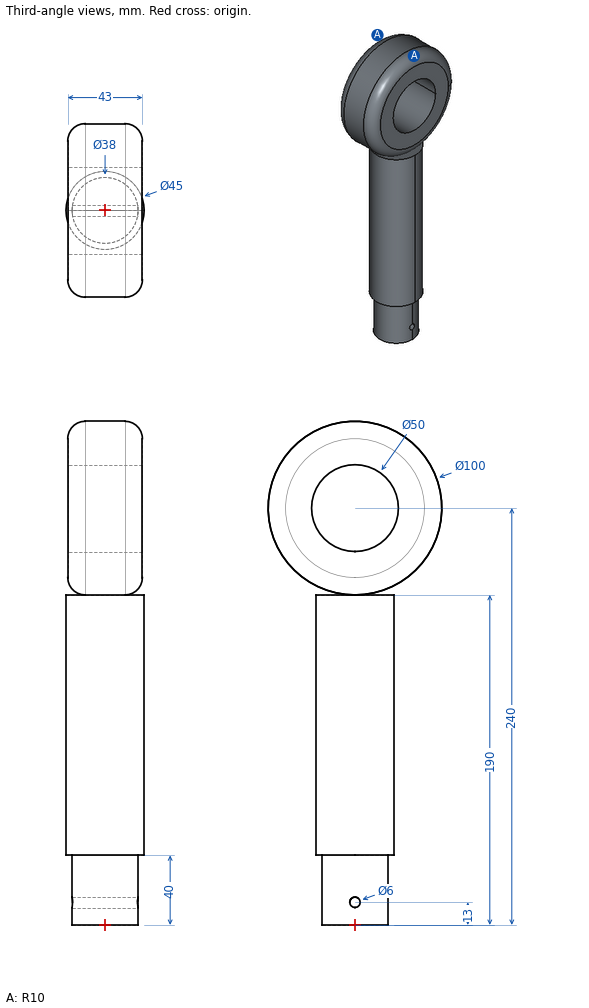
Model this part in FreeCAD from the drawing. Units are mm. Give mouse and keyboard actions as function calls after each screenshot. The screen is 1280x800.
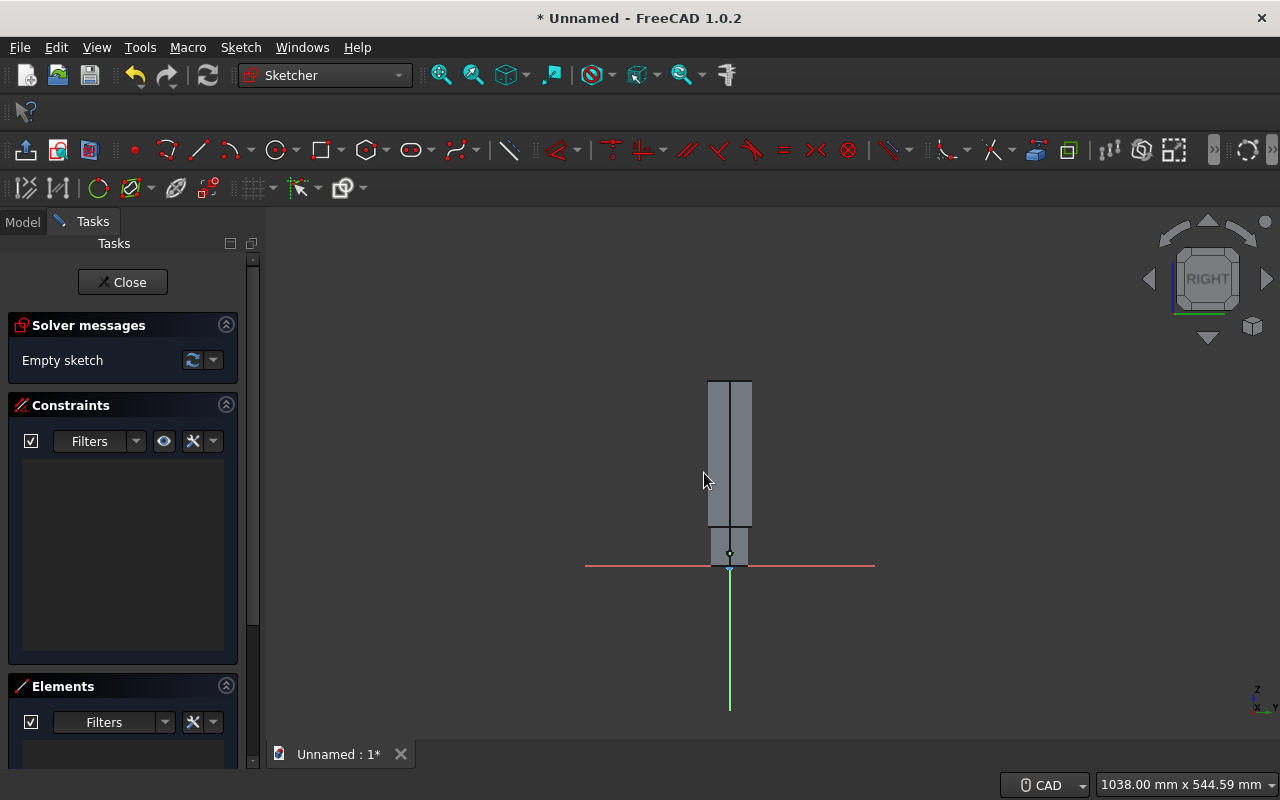
scroll(740, 271, up, 6)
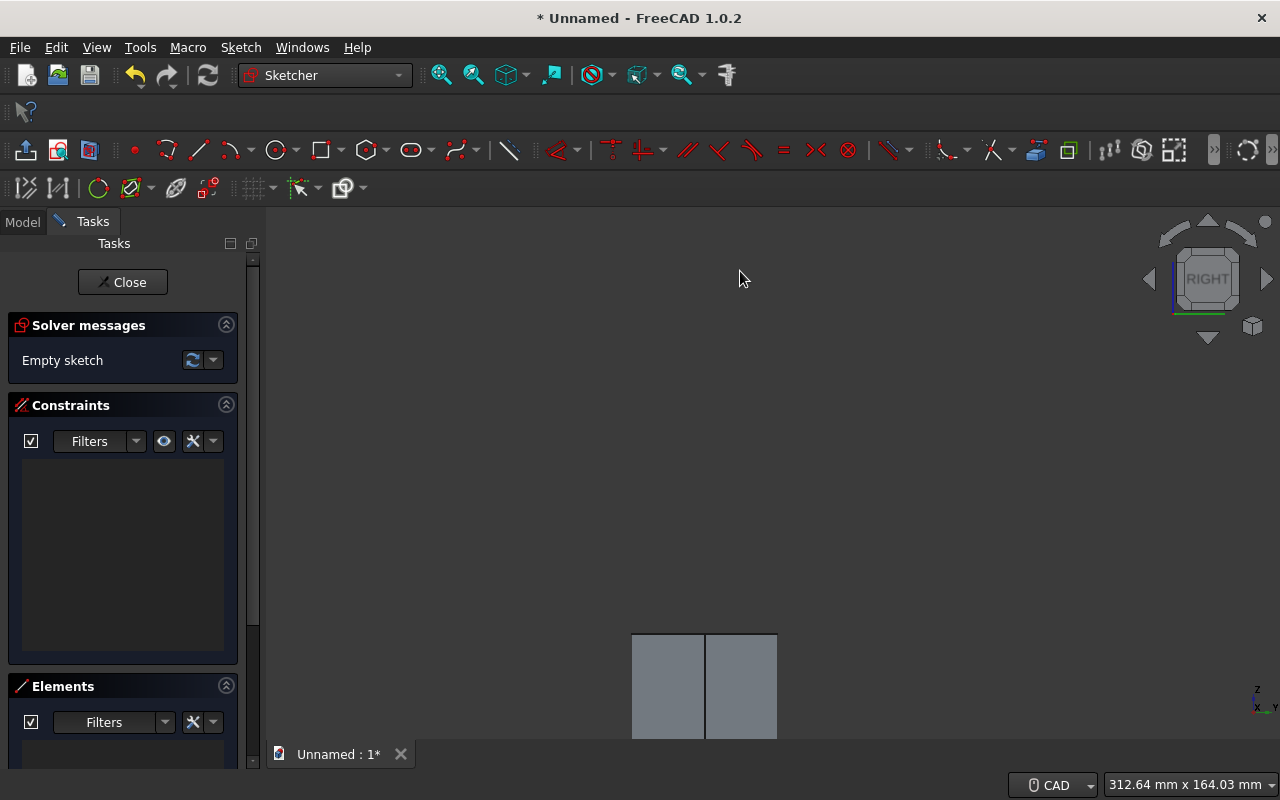
click(276, 150)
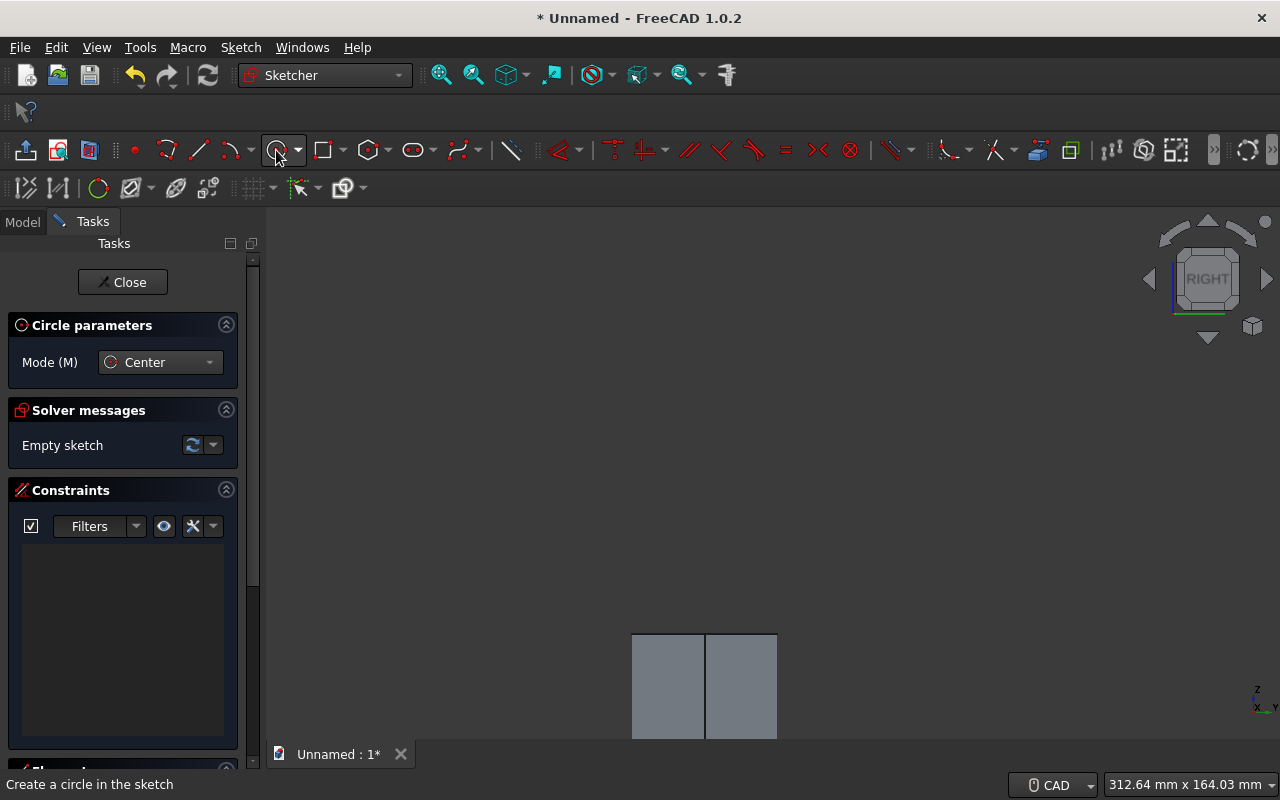
click(705, 472)
move(819, 357)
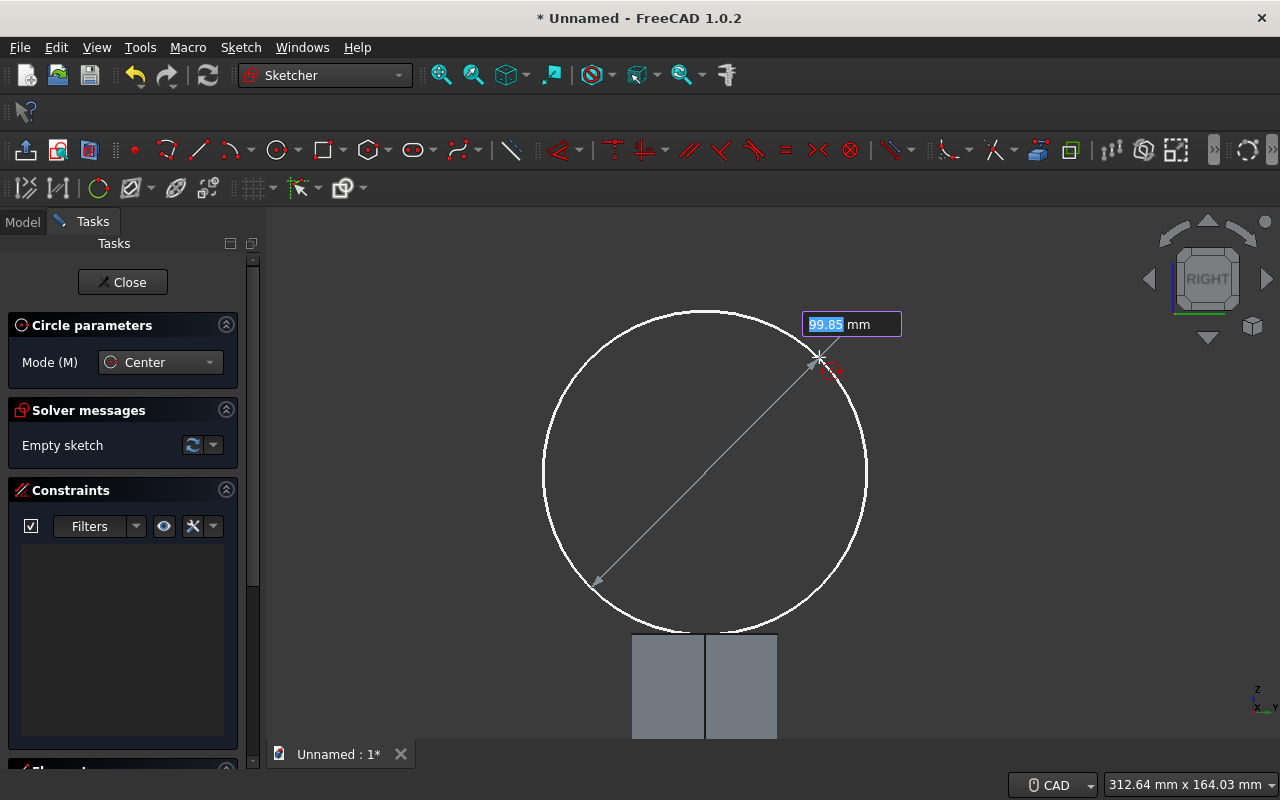
text(100)
key(Return)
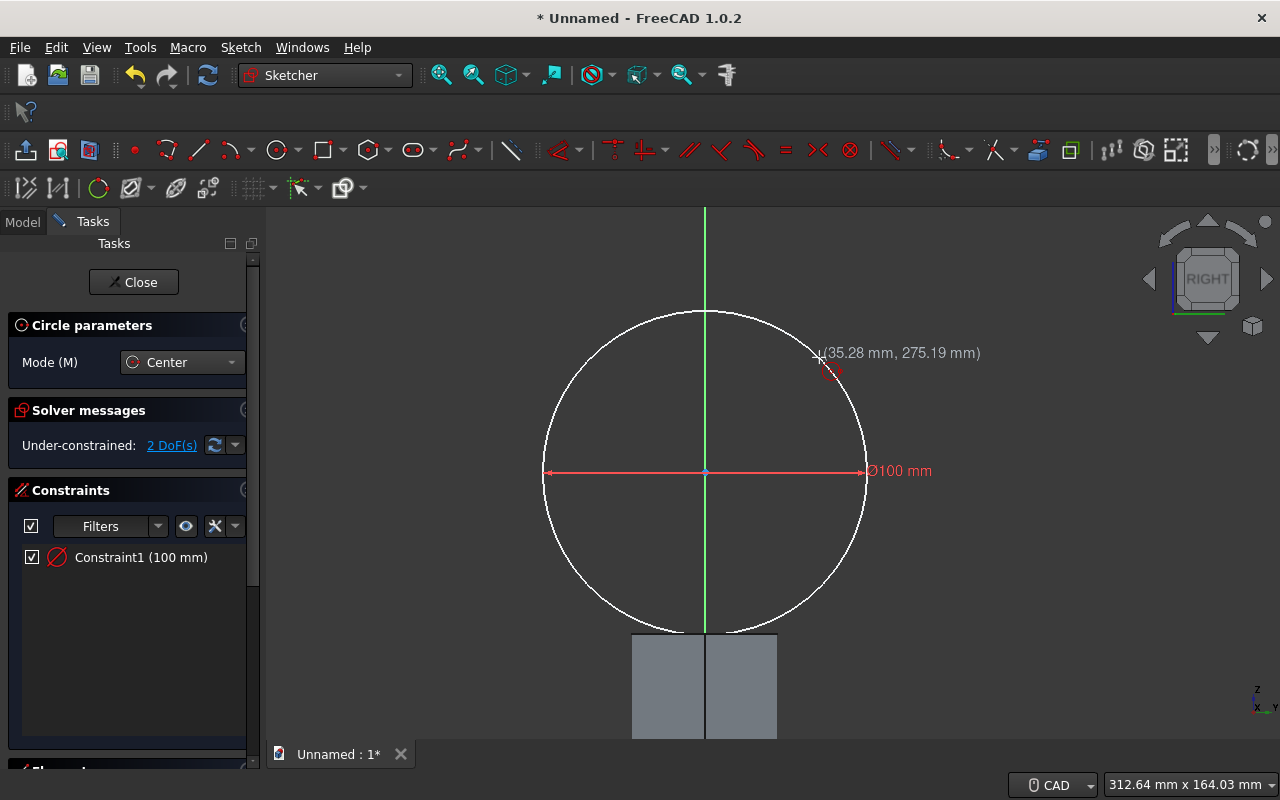
click(705, 473)
move(762, 415)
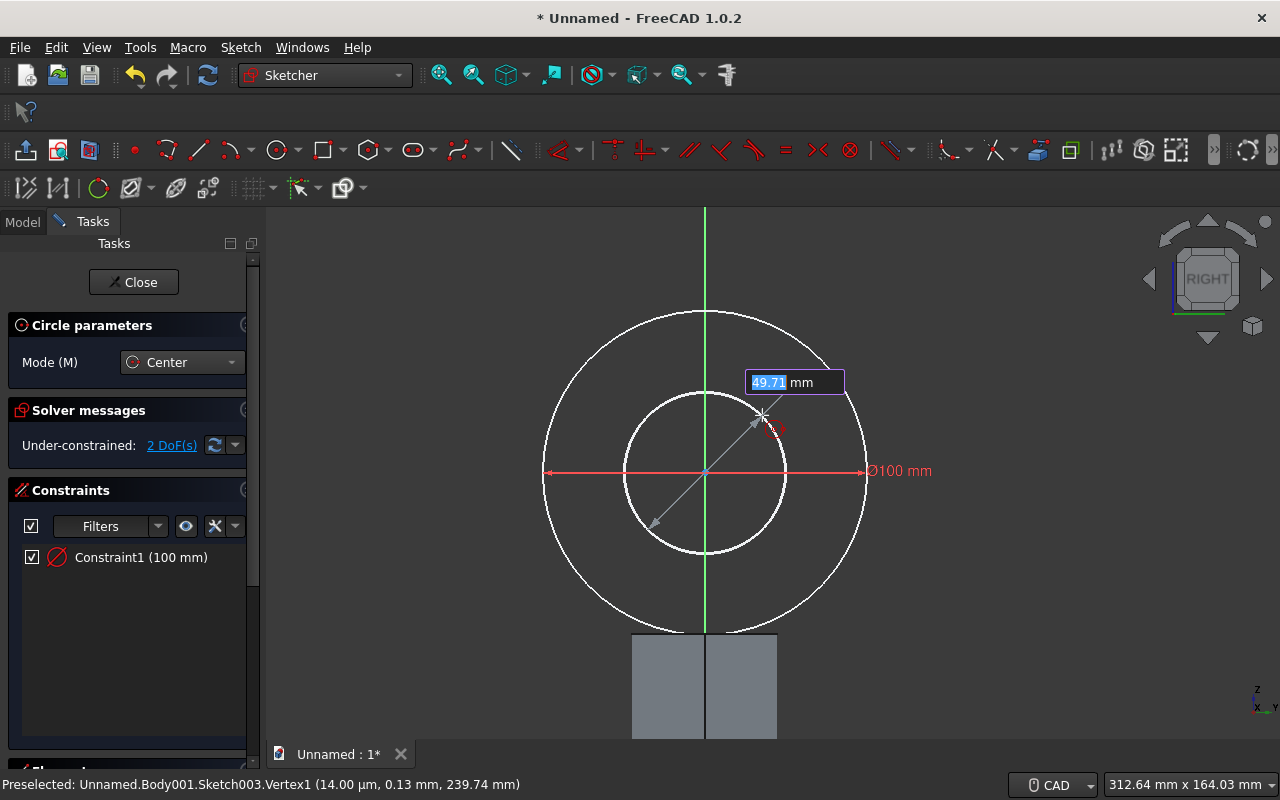
text(50)
key(Return)
key(Escape)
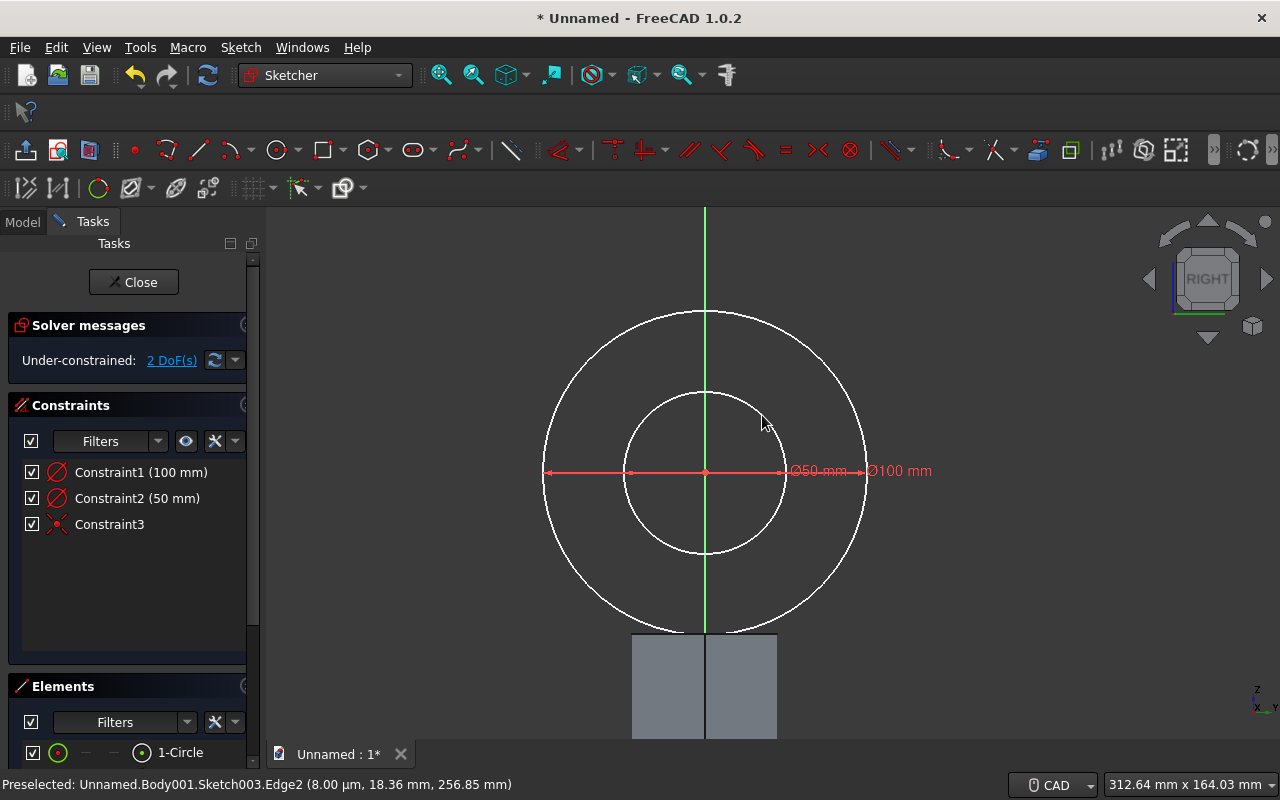
click(705, 473)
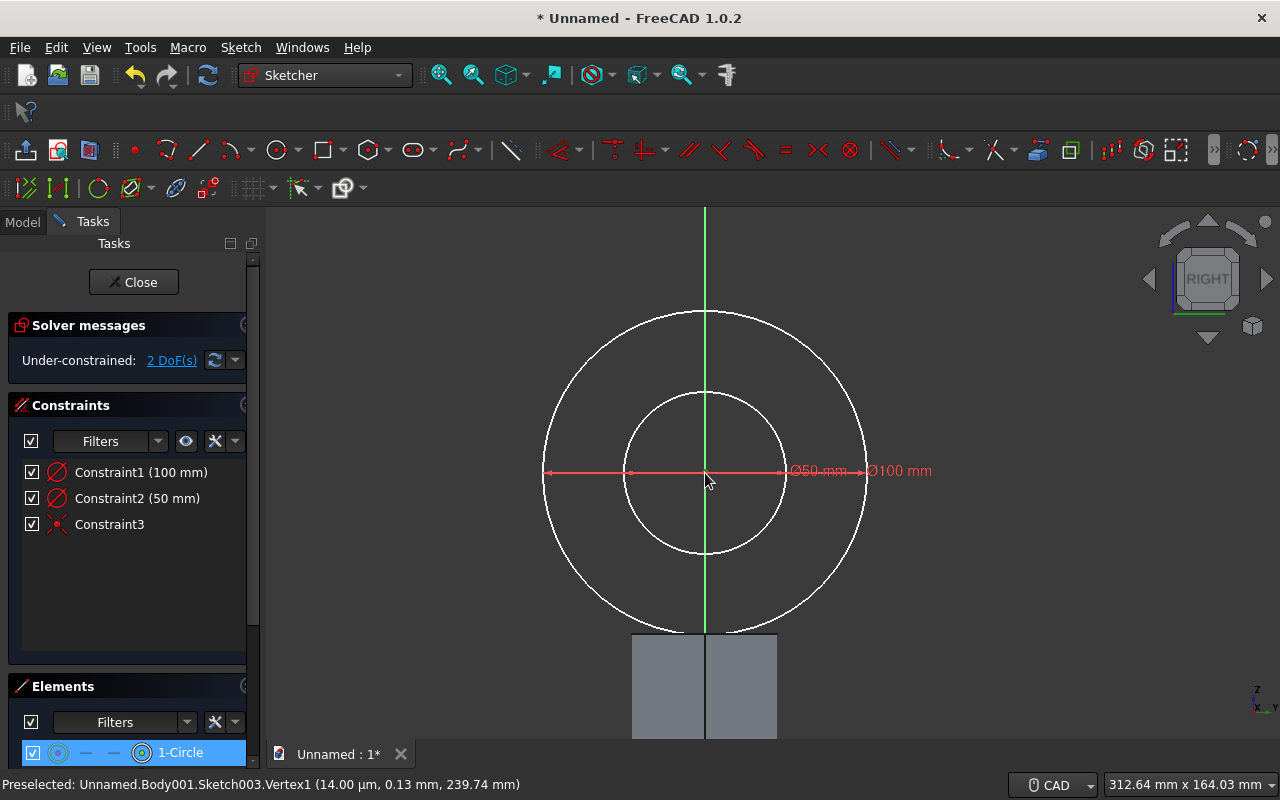
click(705, 677)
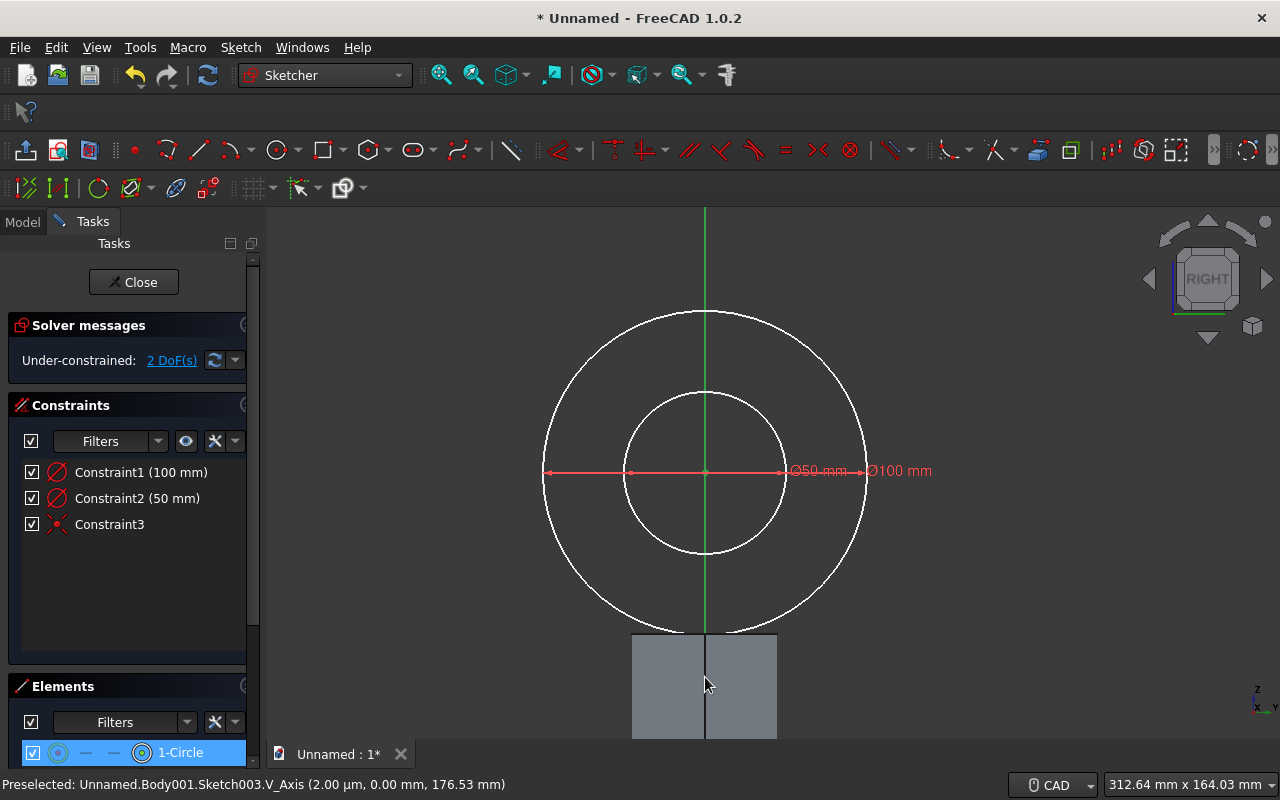
key(c)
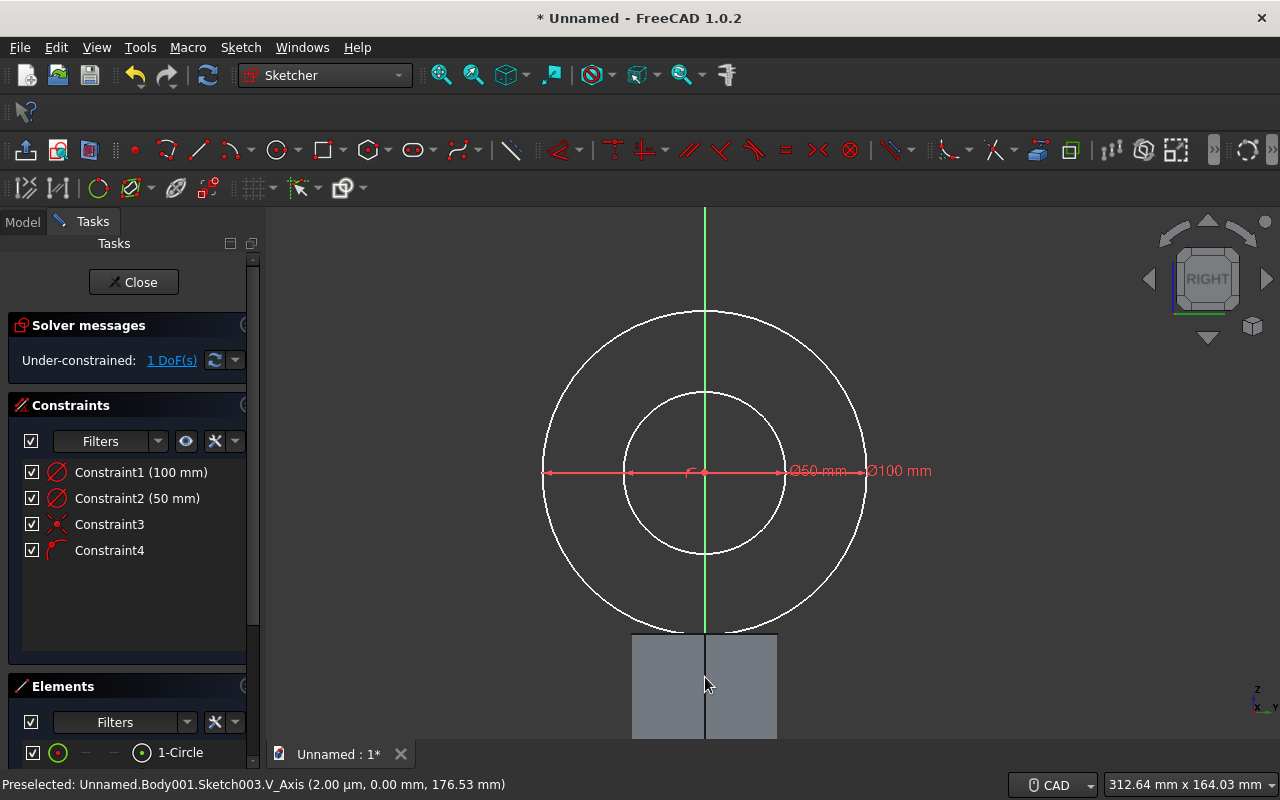
key(d)